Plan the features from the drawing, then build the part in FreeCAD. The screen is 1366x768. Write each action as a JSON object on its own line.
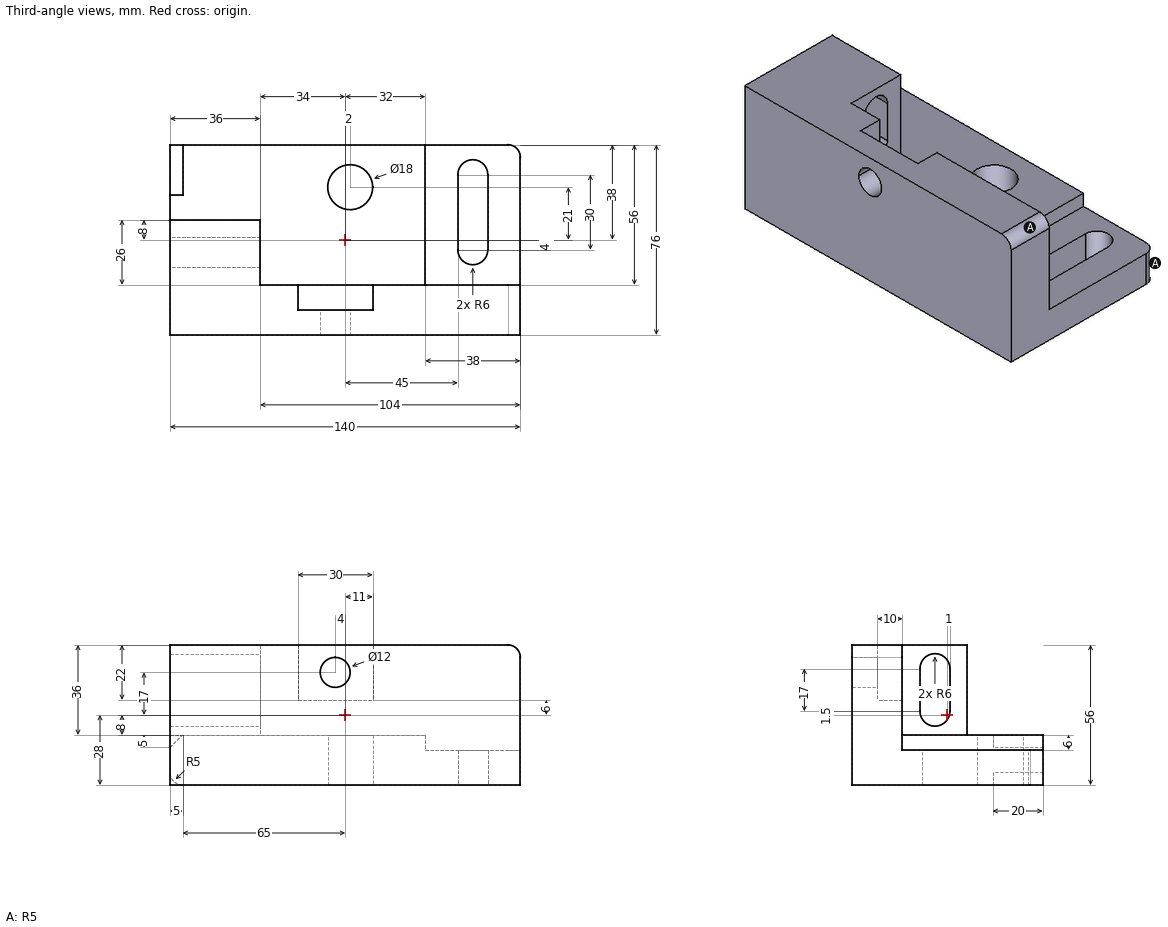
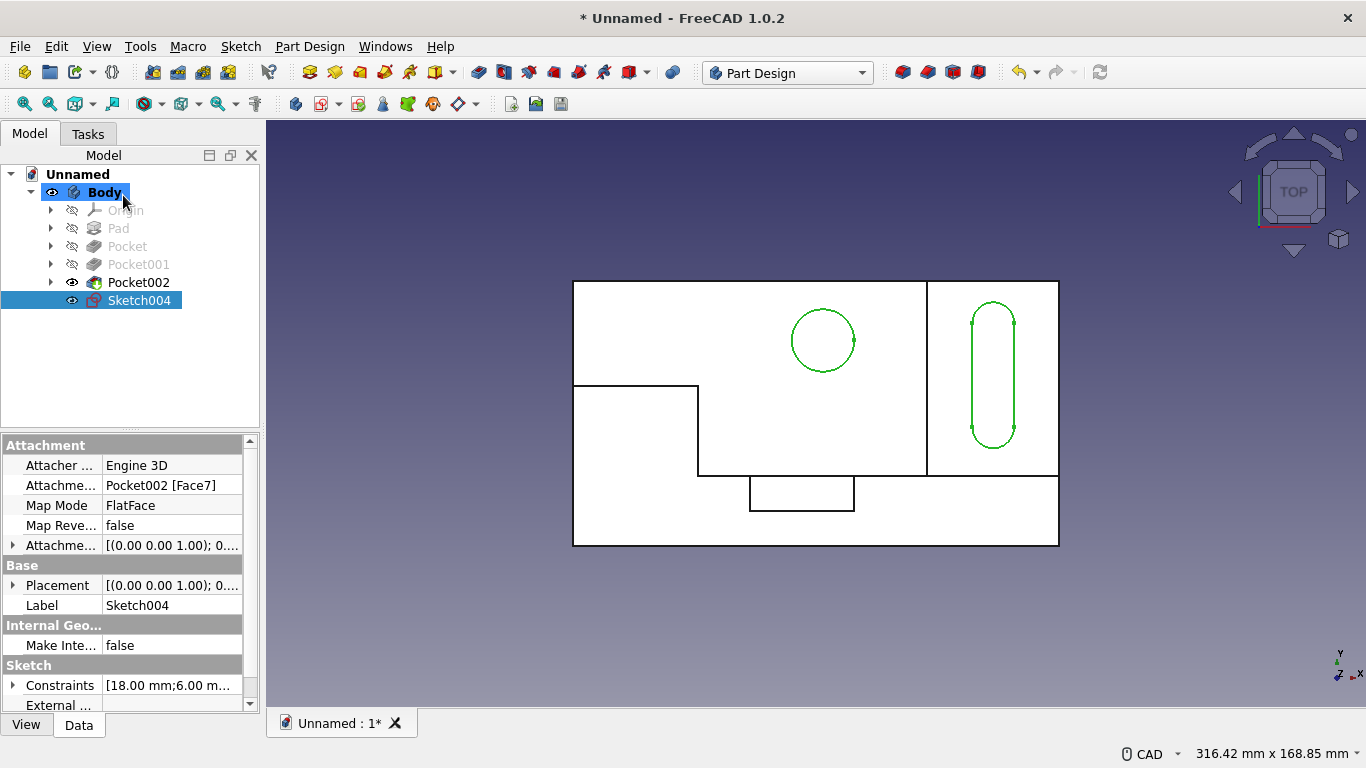
{"action": "left_click", "coordinate": [479, 72]}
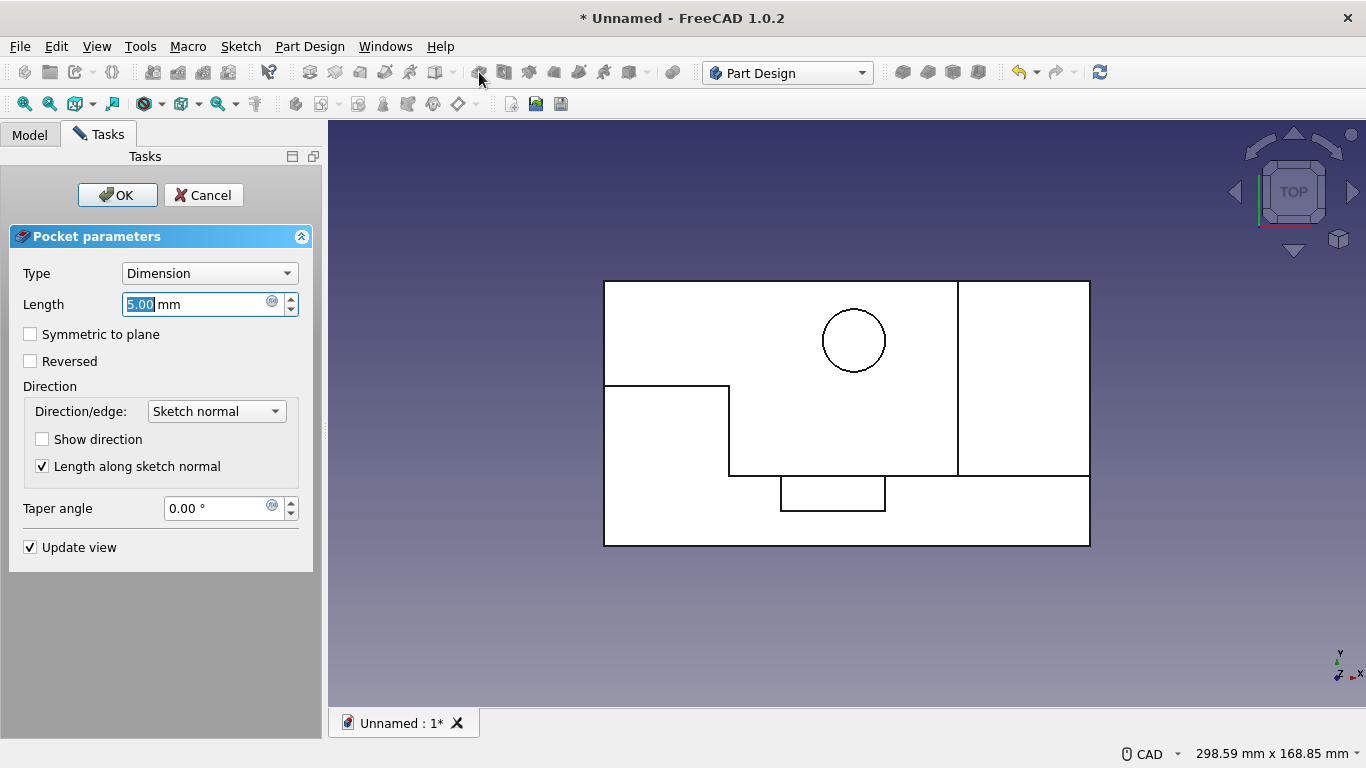
{"action": "left_click", "coordinate": [210, 274]}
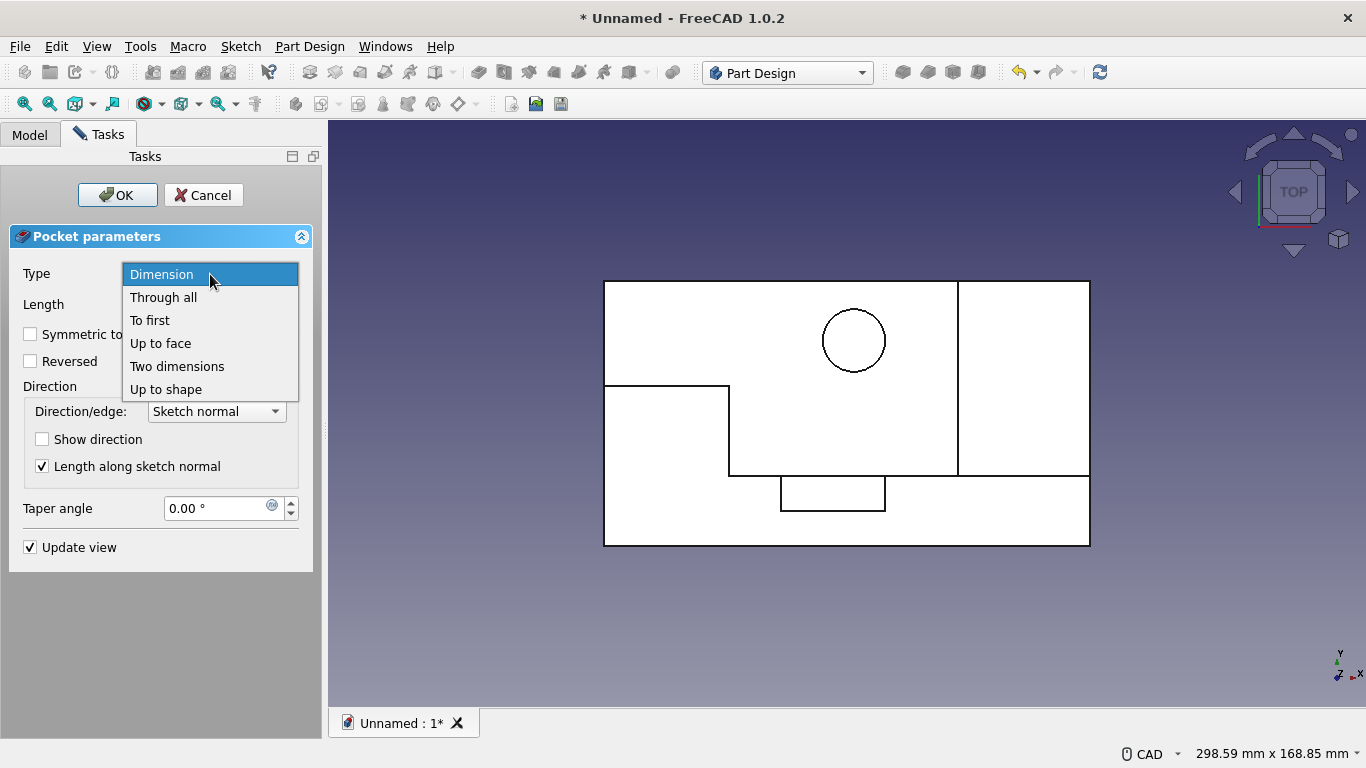
{"action": "left_click", "coordinate": [208, 298]}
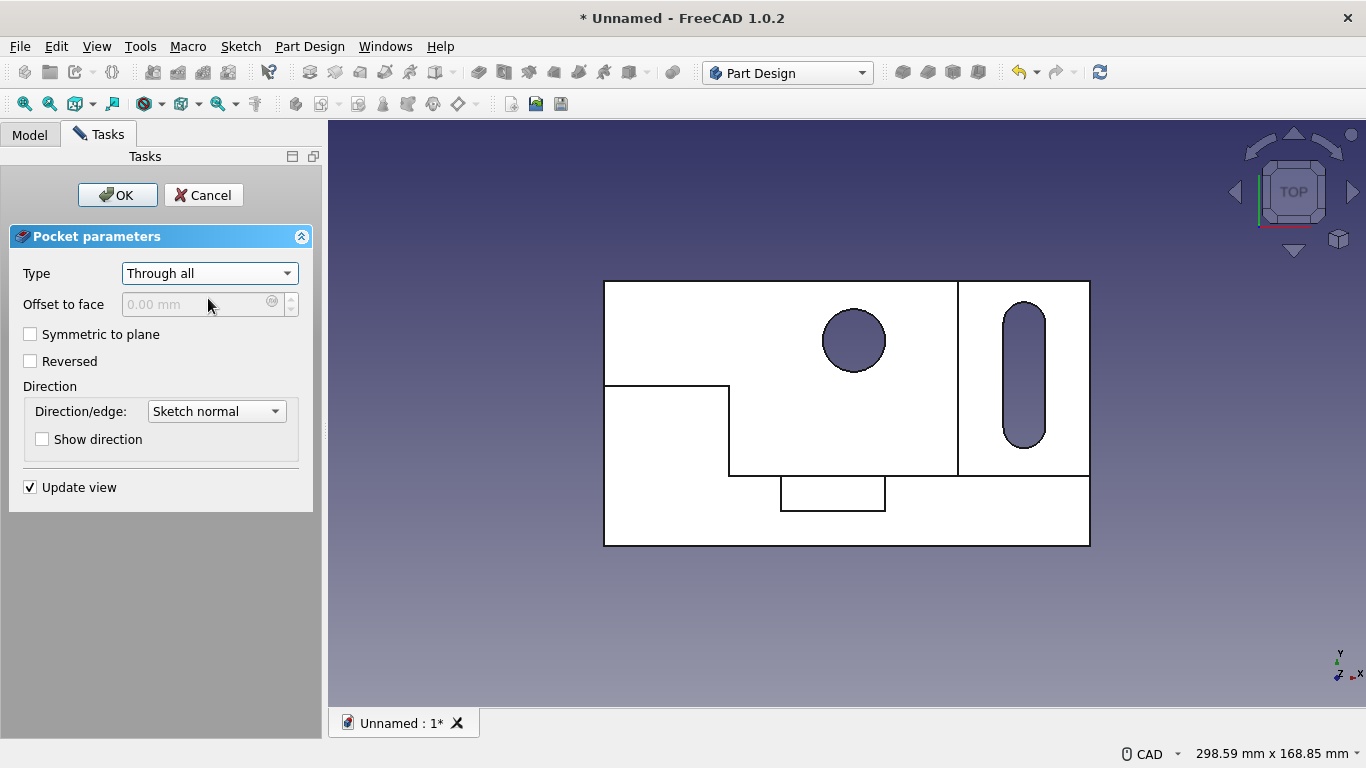
{"action": "left_click", "coordinate": [118, 195]}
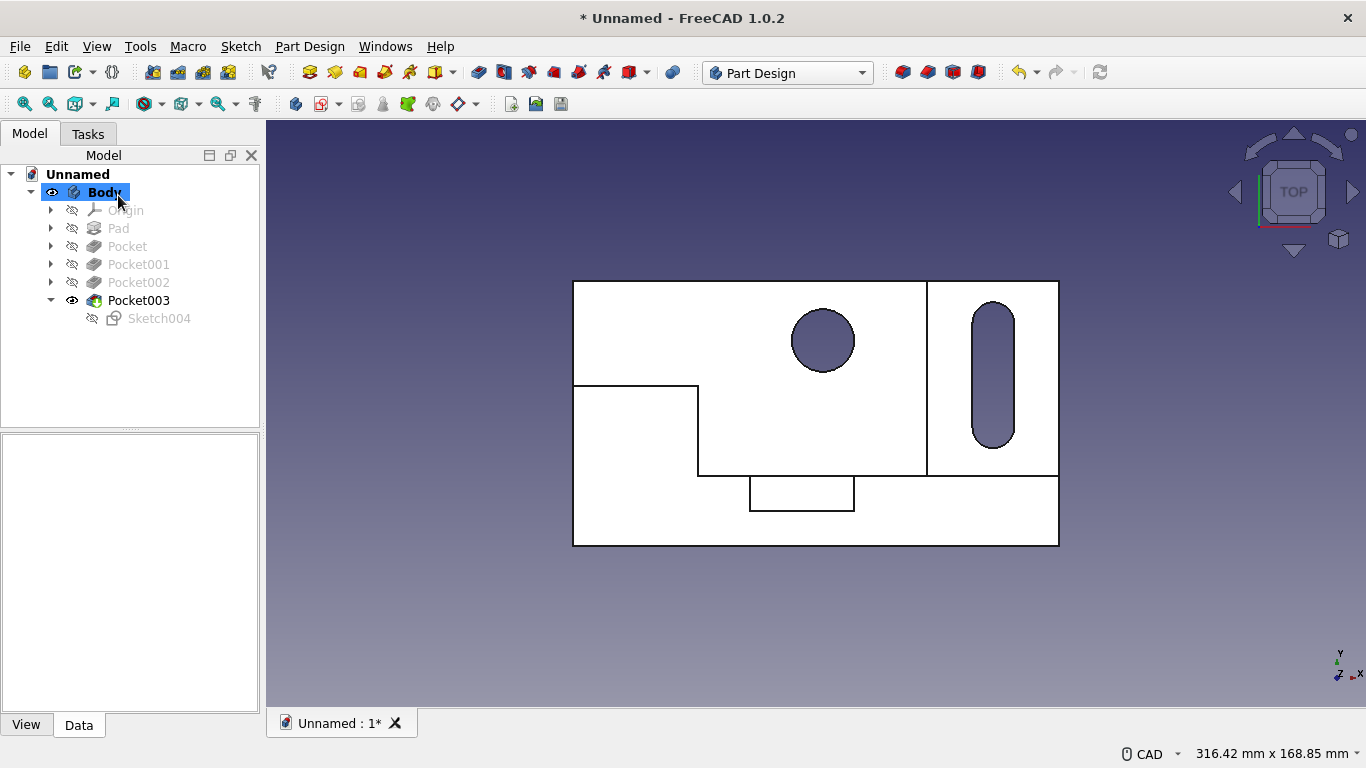
{"action": "key", "text": "4"}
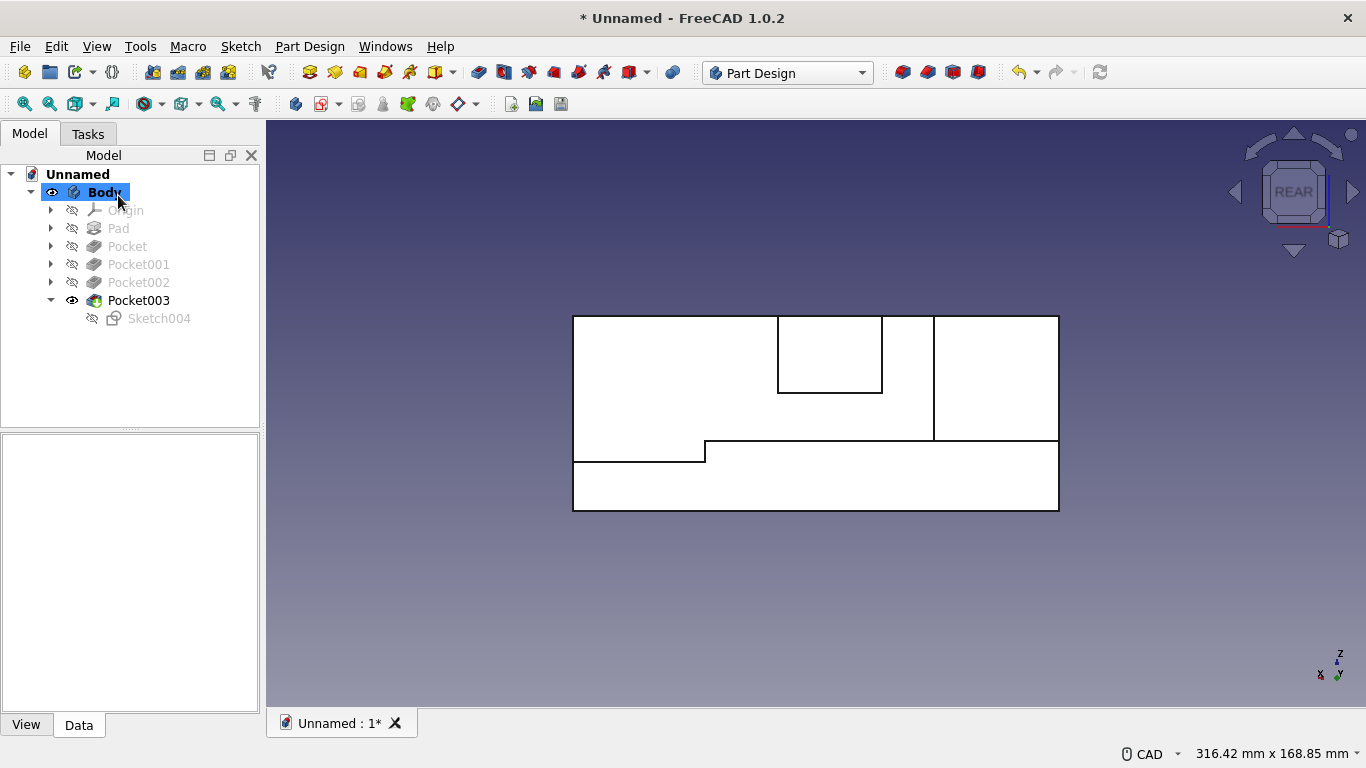
{"action": "left_click", "coordinate": [25, 104]}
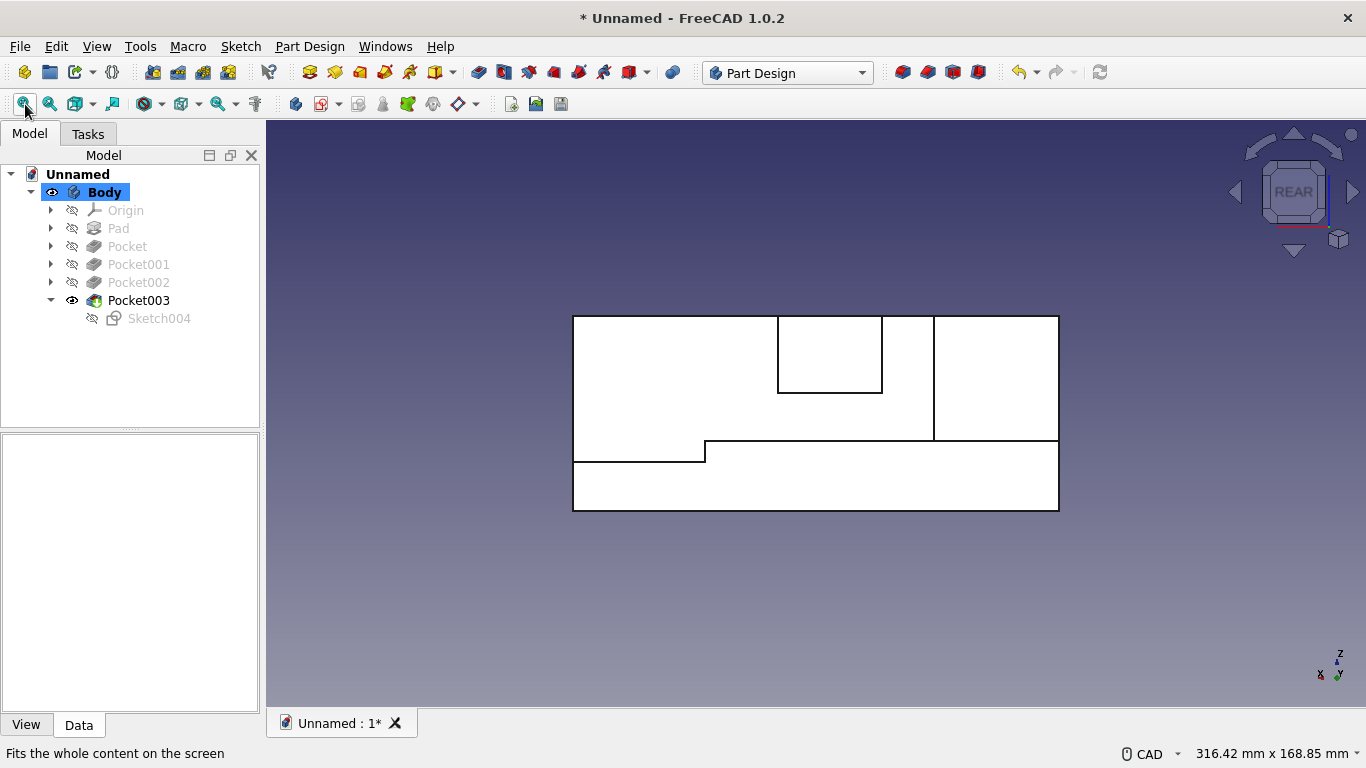
{"action": "left_click", "coordinate": [746, 475]}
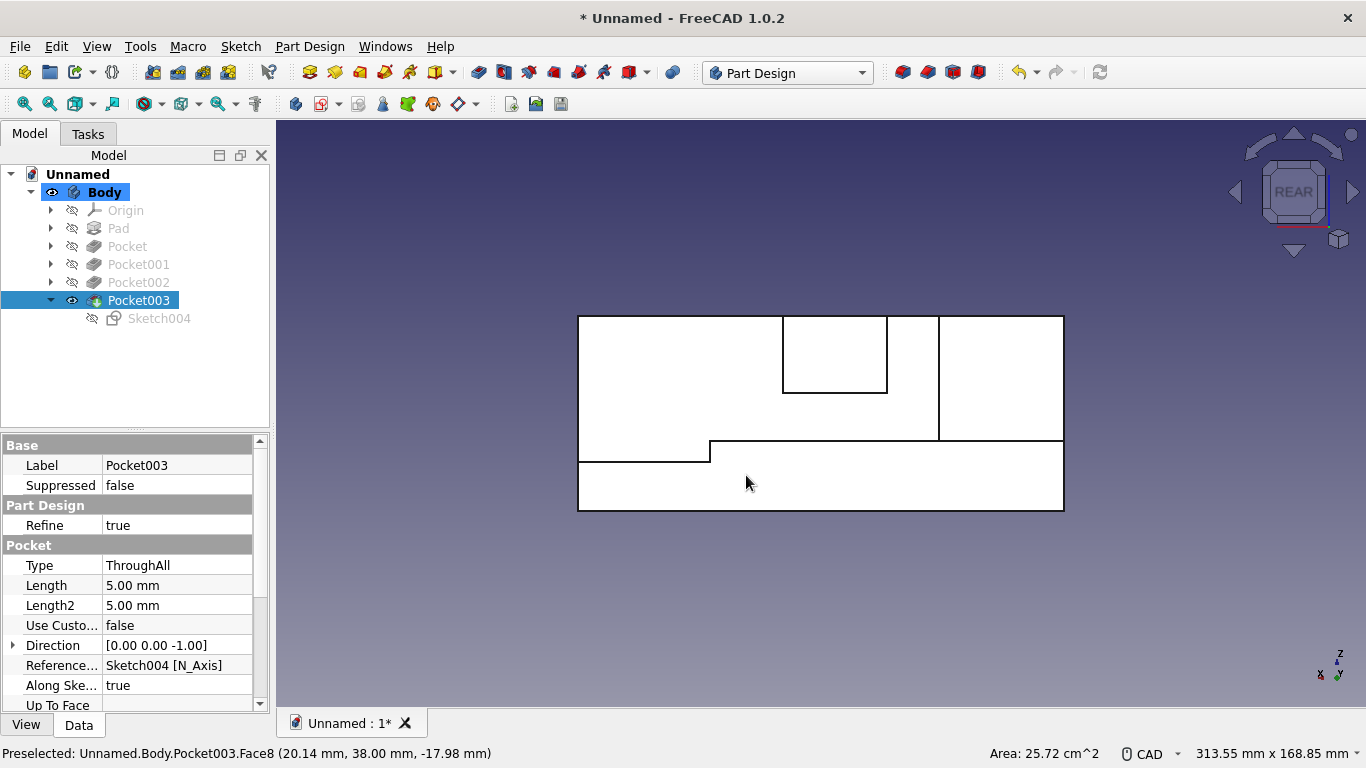
{"action": "left_click", "coordinate": [320, 104]}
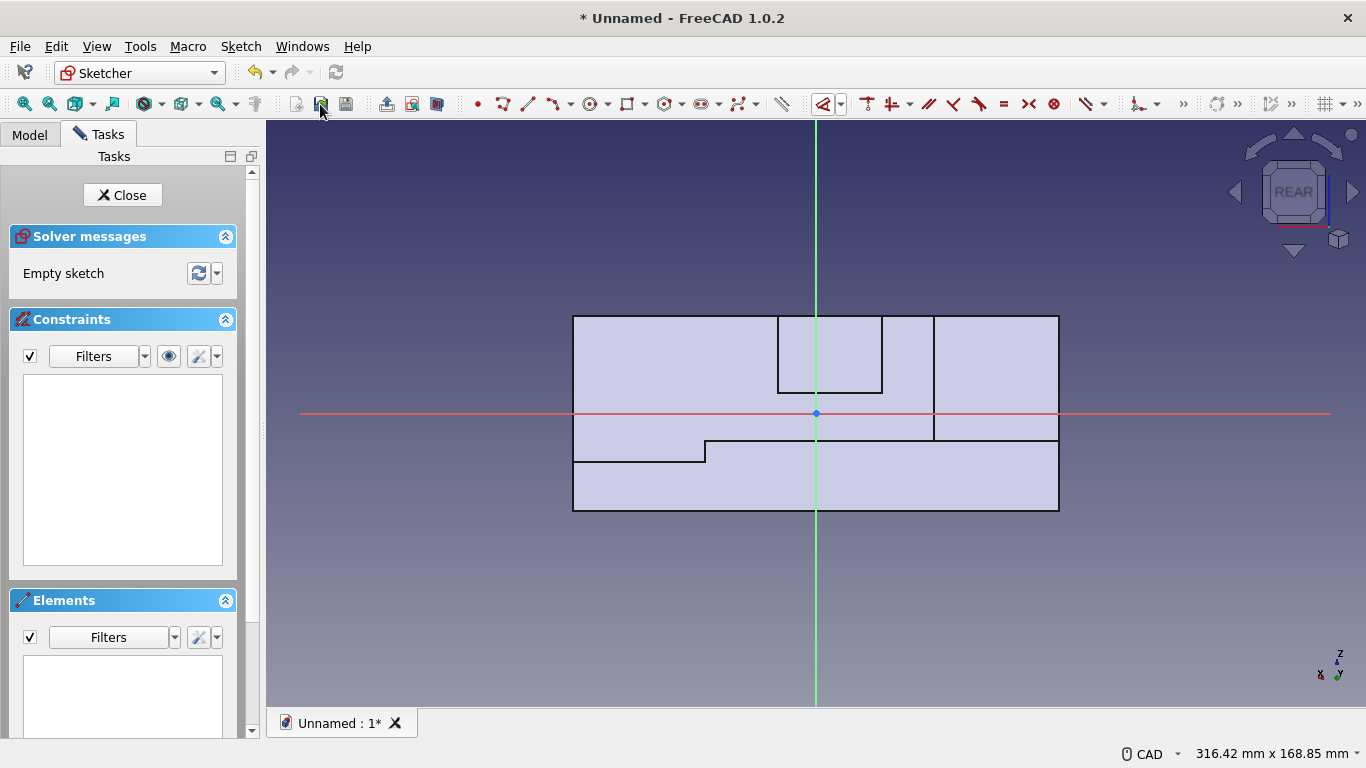
{"action": "scroll", "coordinate": [1127, 492], "scroll_direction": "up", "scroll_amount": 8}